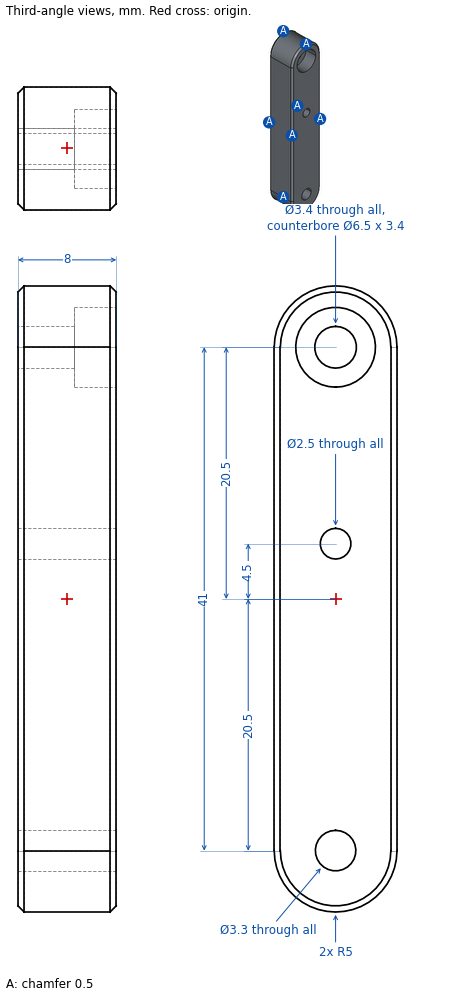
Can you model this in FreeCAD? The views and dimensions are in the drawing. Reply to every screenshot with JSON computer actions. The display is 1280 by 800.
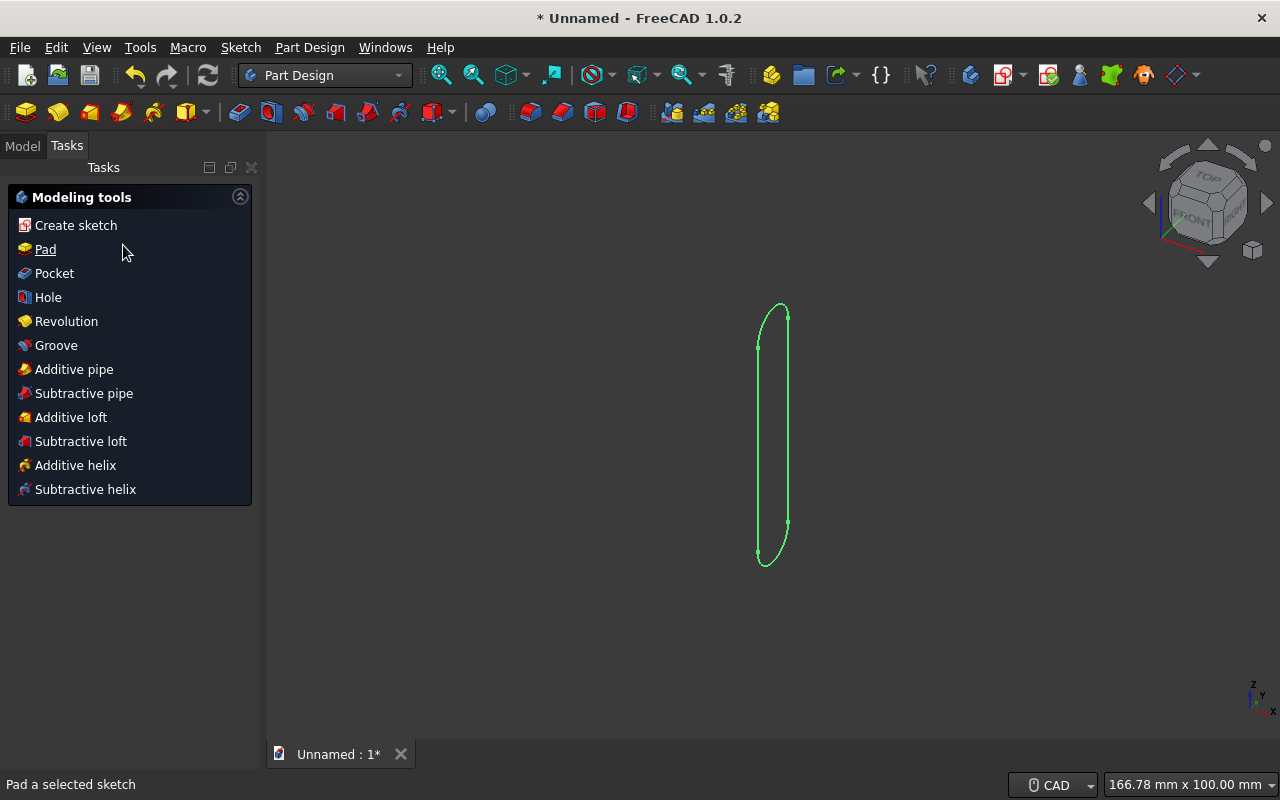
{"action": "left_click", "coordinate": [26, 112]}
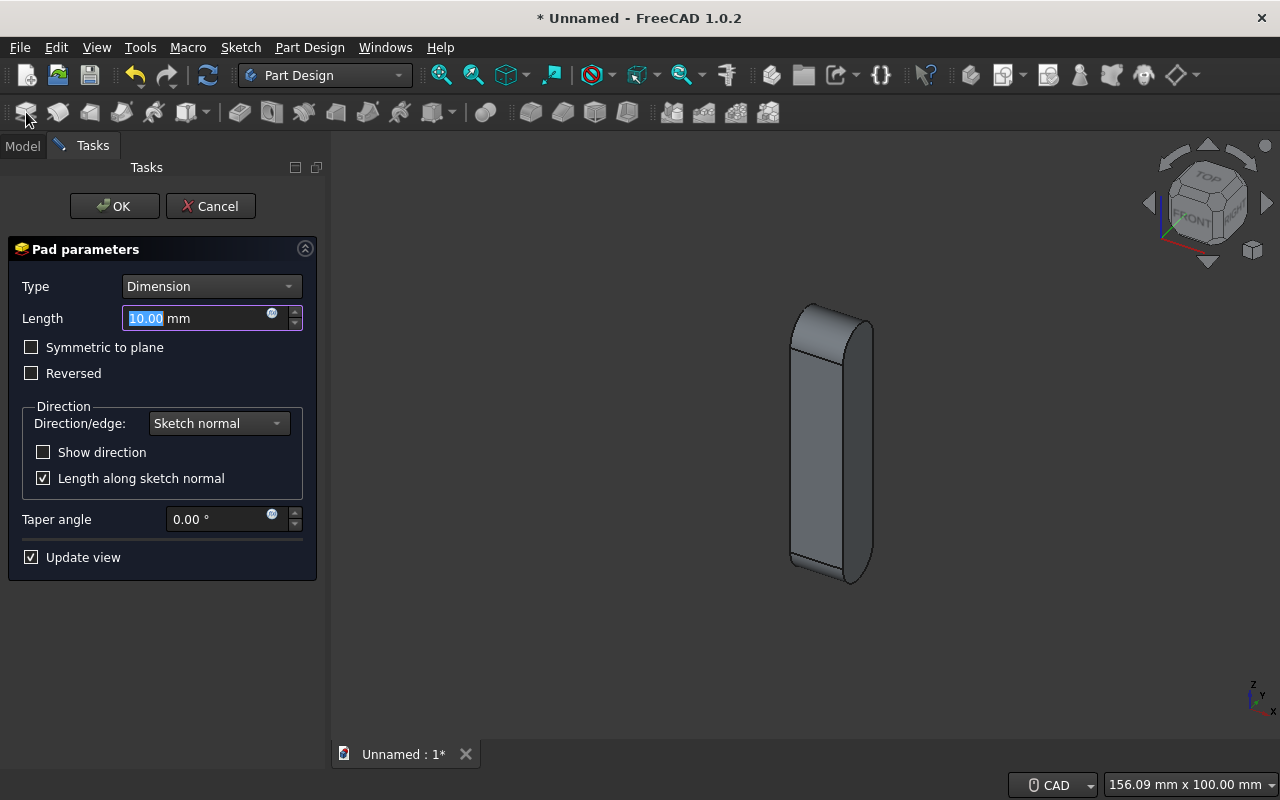
{"action": "type", "text": "8"}
{"action": "key", "text": "Tab"}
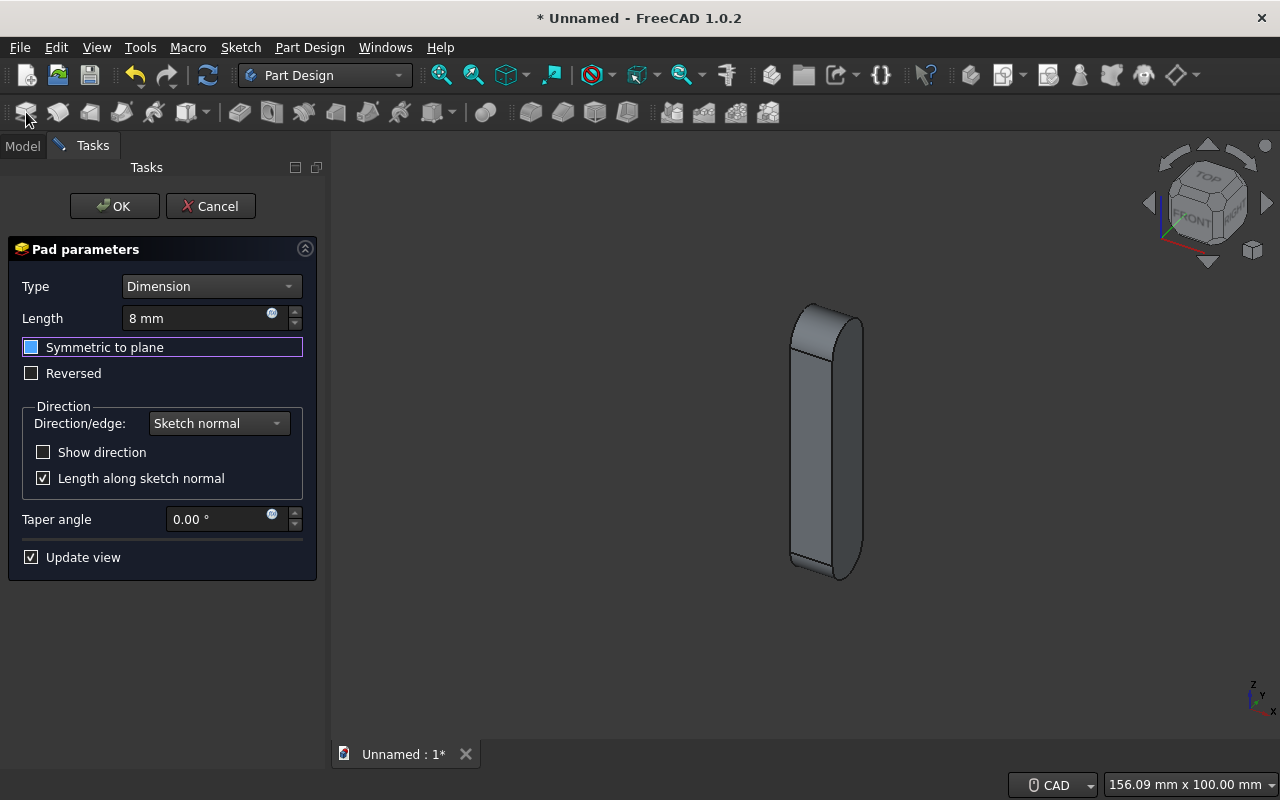
{"action": "left_click", "coordinate": [30, 347]}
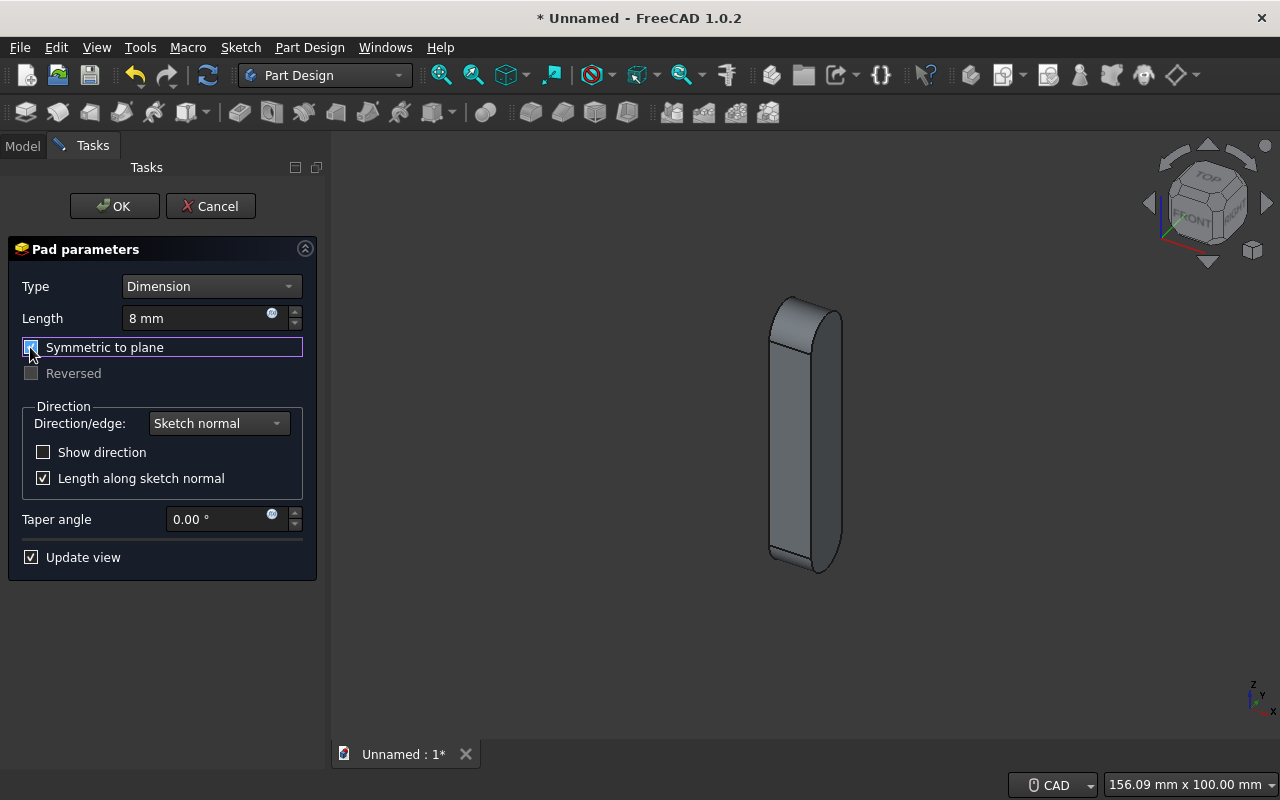
{"action": "left_click", "coordinate": [115, 206]}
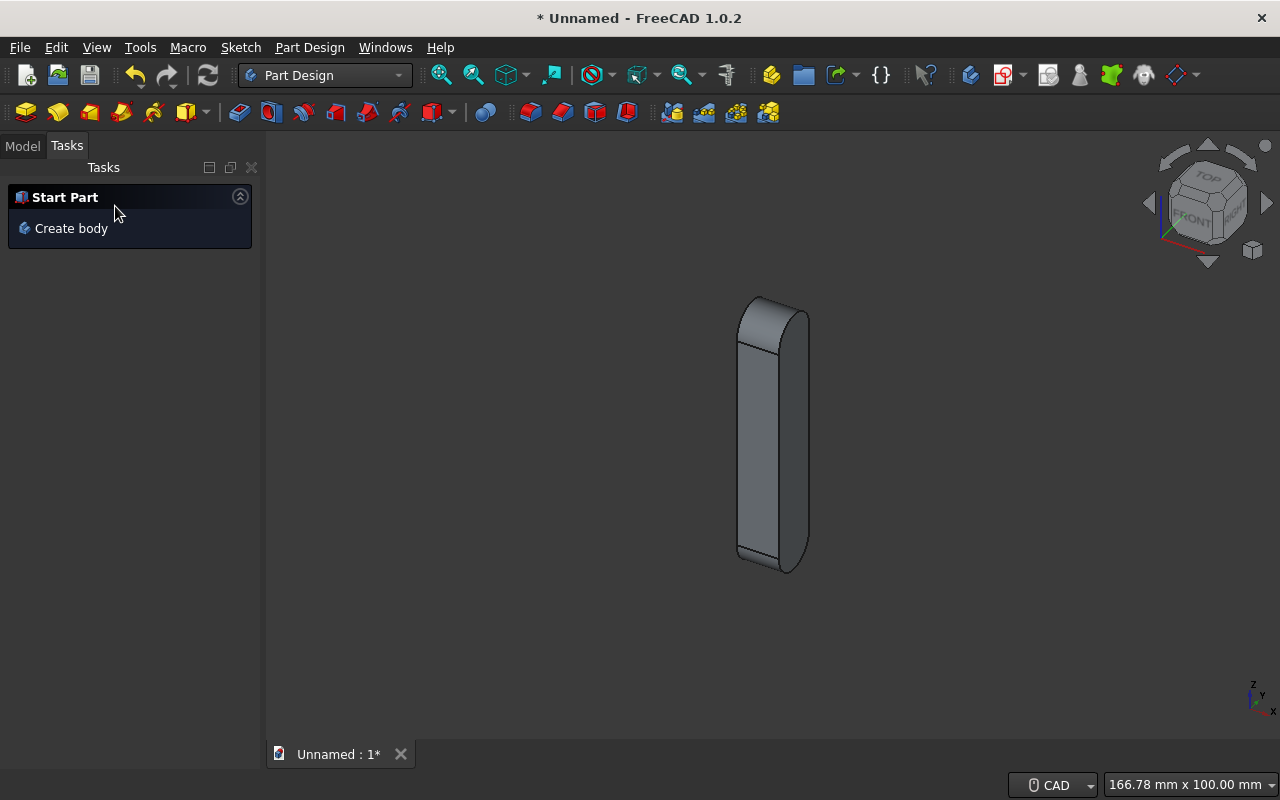
{"action": "left_click", "coordinate": [794, 514]}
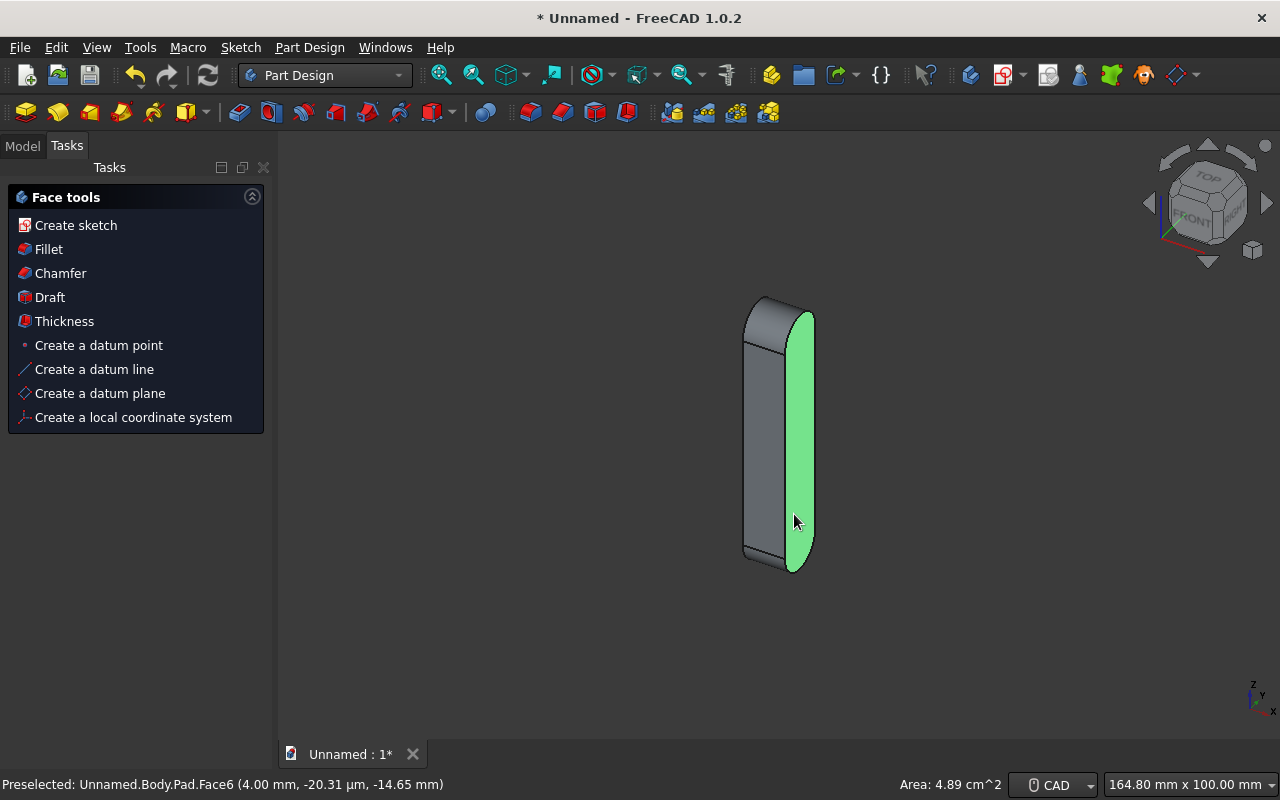
{"action": "left_click", "coordinate": [1004, 76]}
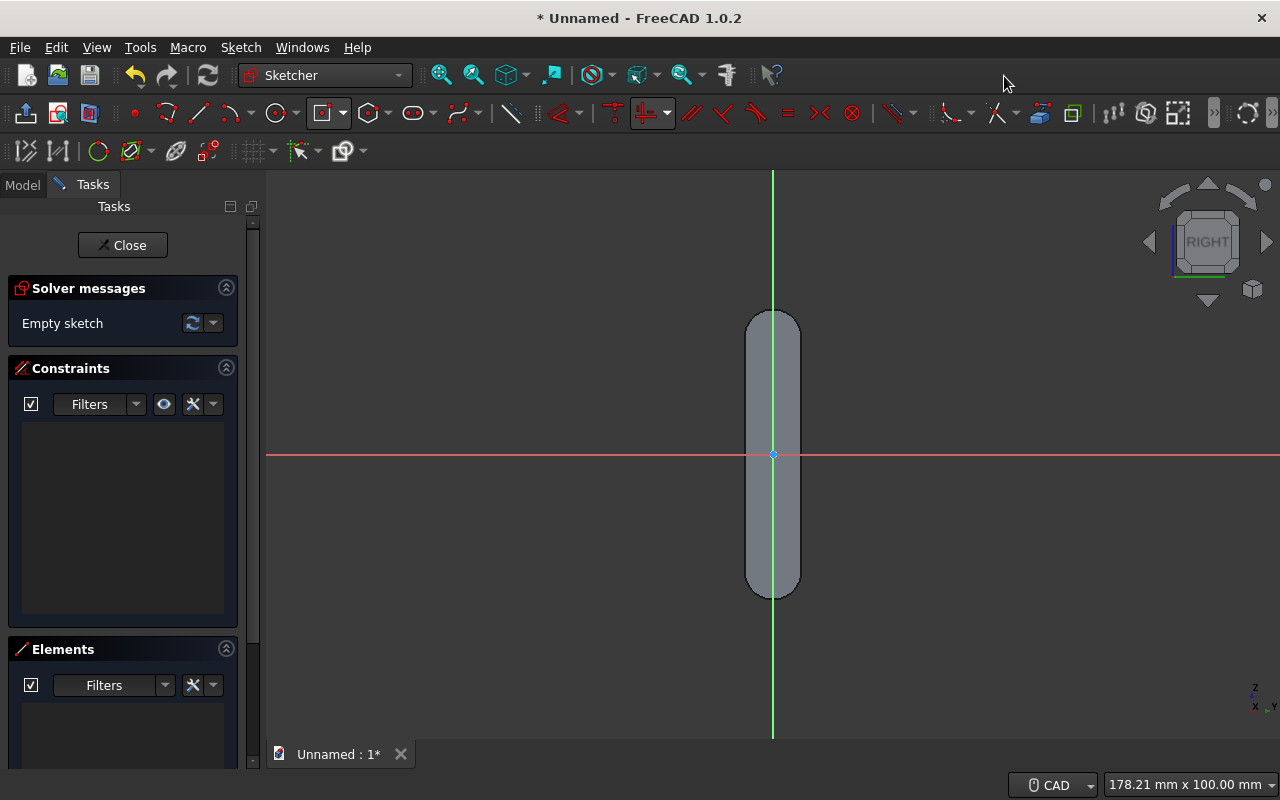
{"action": "scroll", "coordinate": [777, 332], "scroll_direction": "up", "scroll_amount": 15}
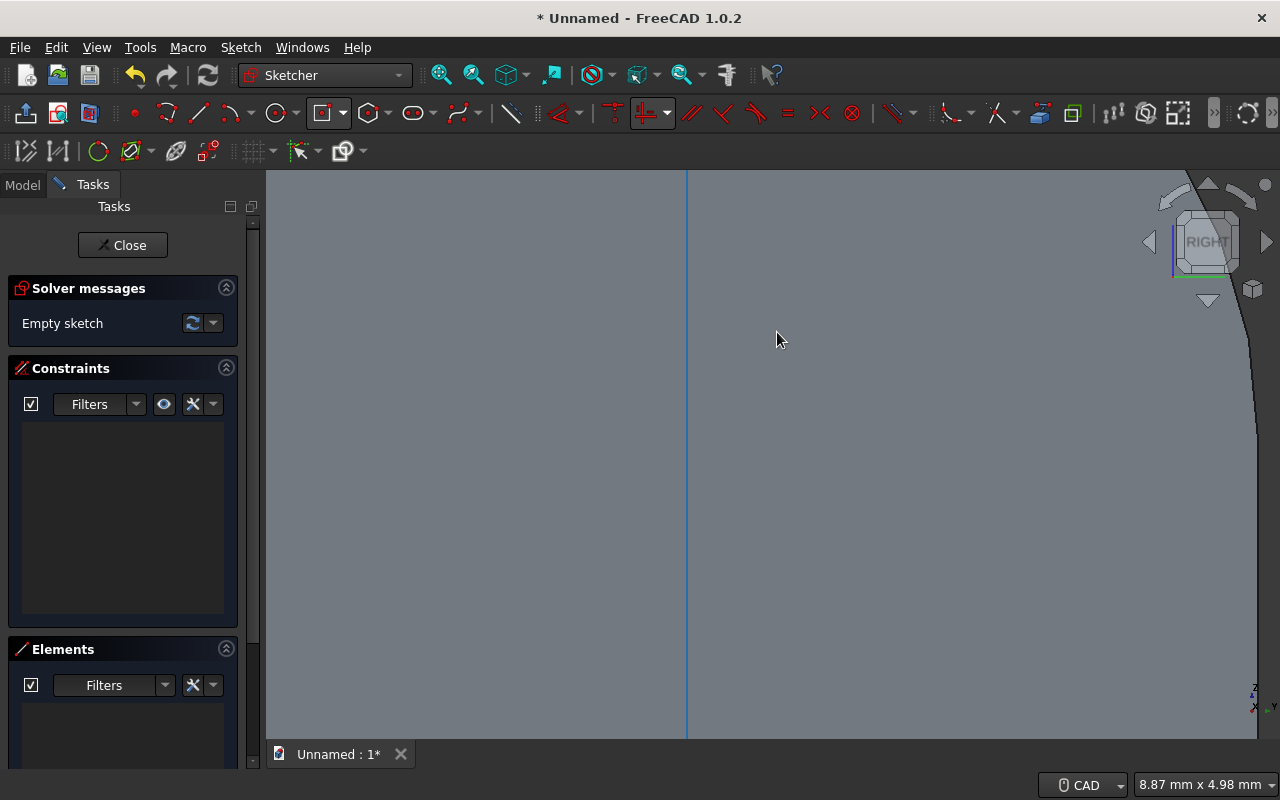
{"action": "key", "text": "g c"}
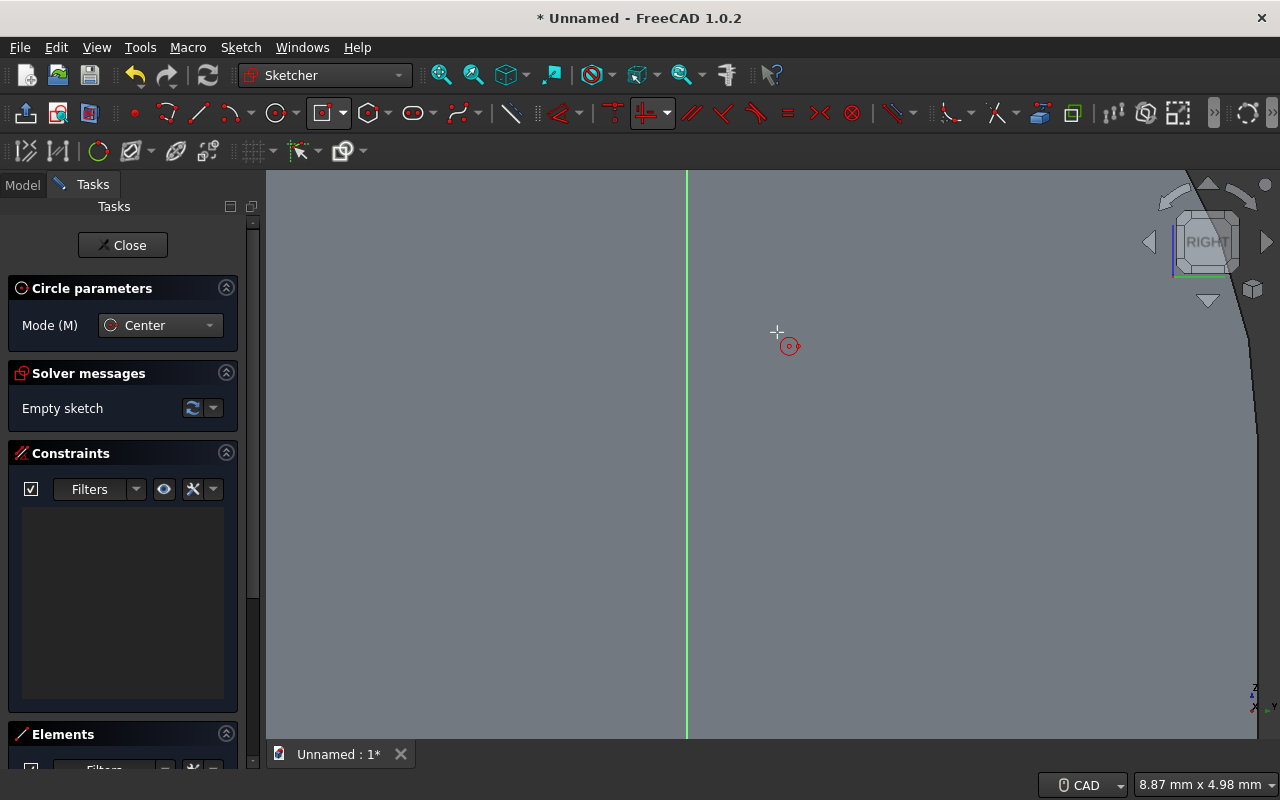
{"action": "left_click", "coordinate": [687, 444]}
{"action": "left_click", "coordinate": [824, 307]}
{"action": "key", "text": "Escape"}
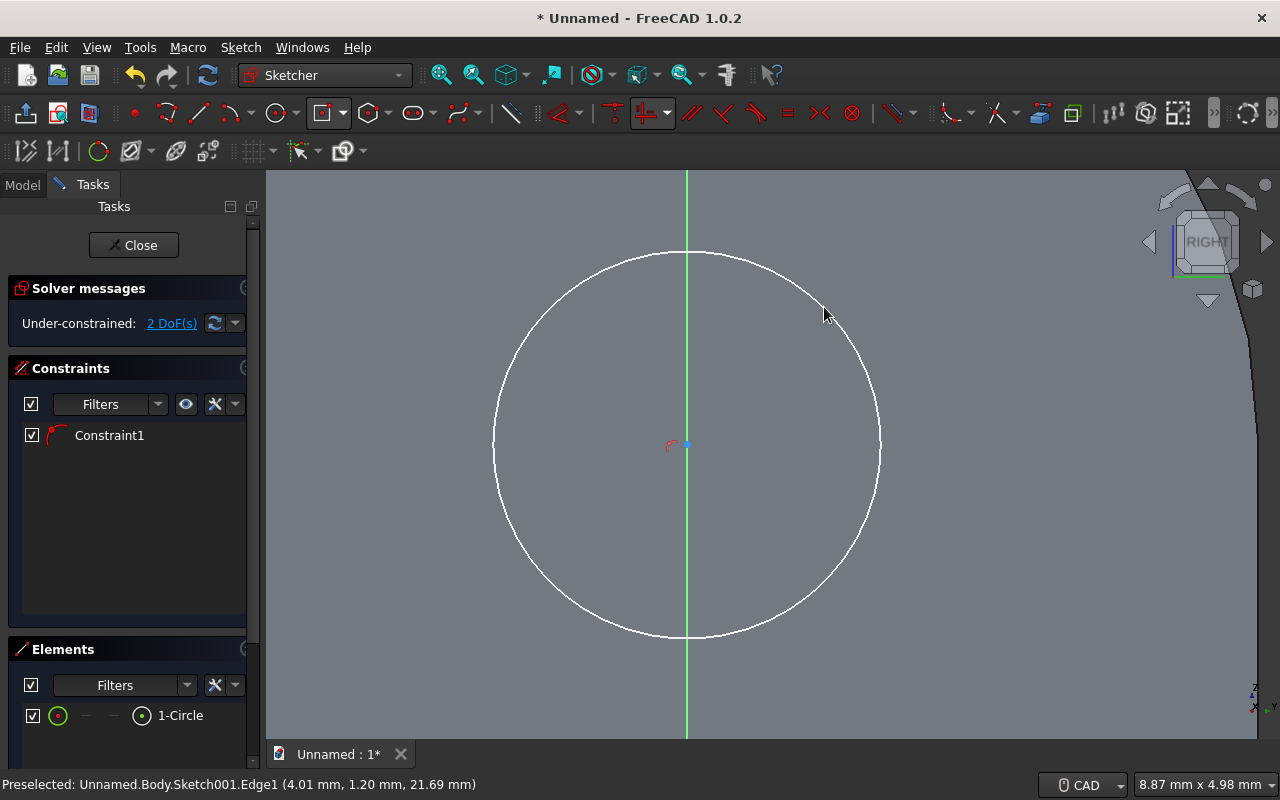
{"action": "key", "text": "d"}